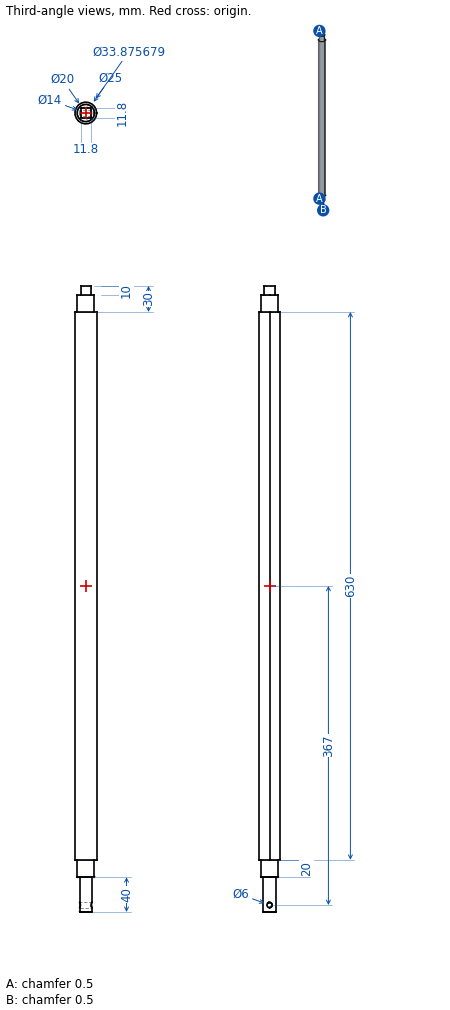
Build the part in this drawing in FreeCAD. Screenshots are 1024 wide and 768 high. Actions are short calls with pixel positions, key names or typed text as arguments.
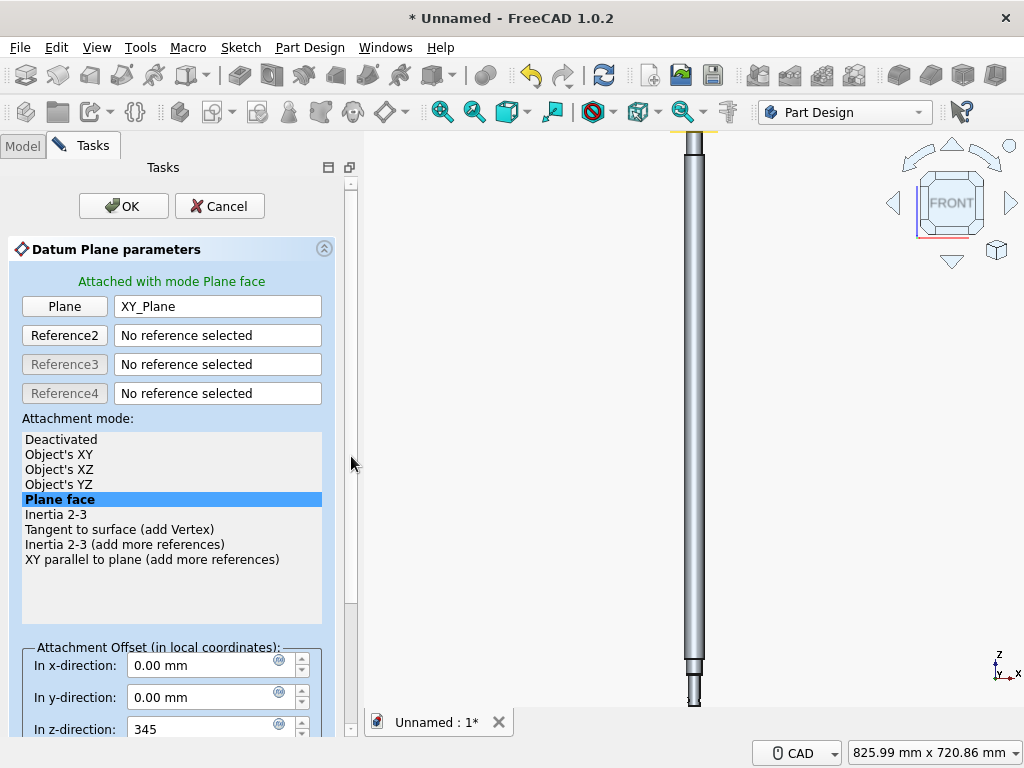
click(124, 206)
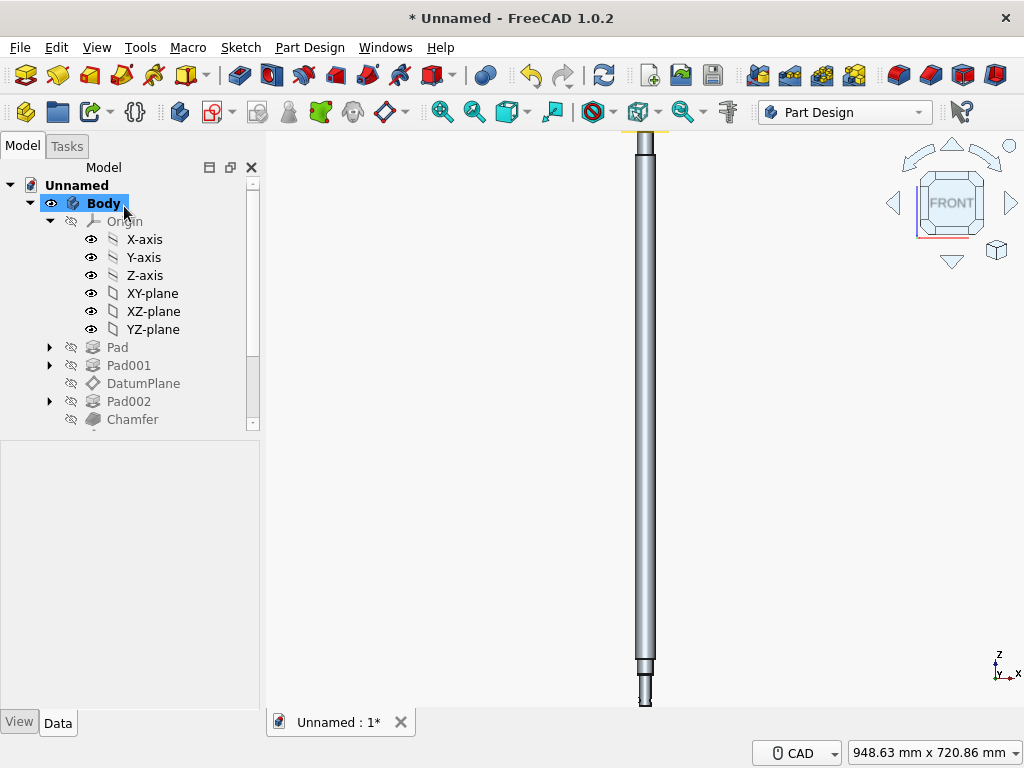
scroll(100, 307, down, 3)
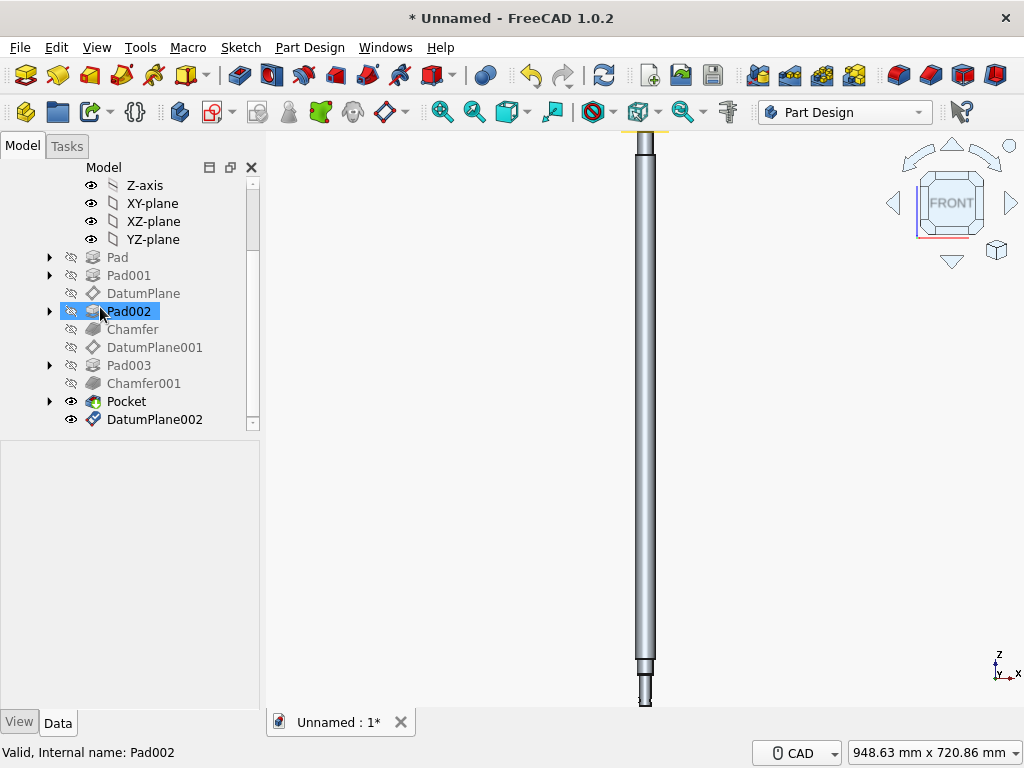
click(116, 419)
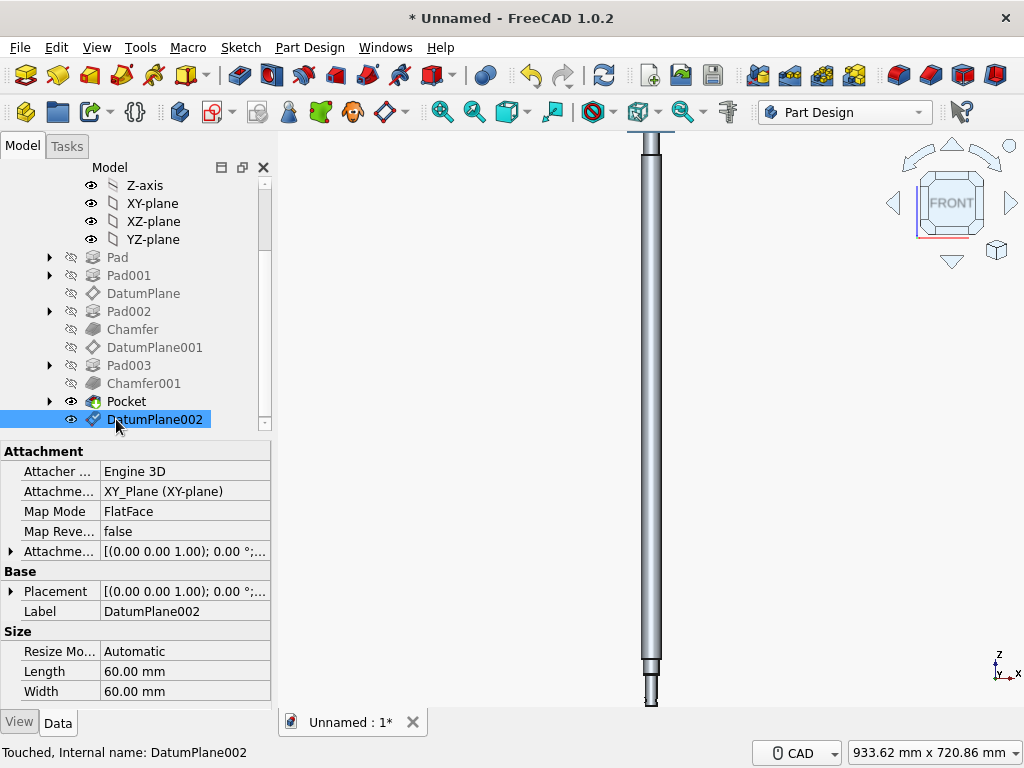
click(212, 112)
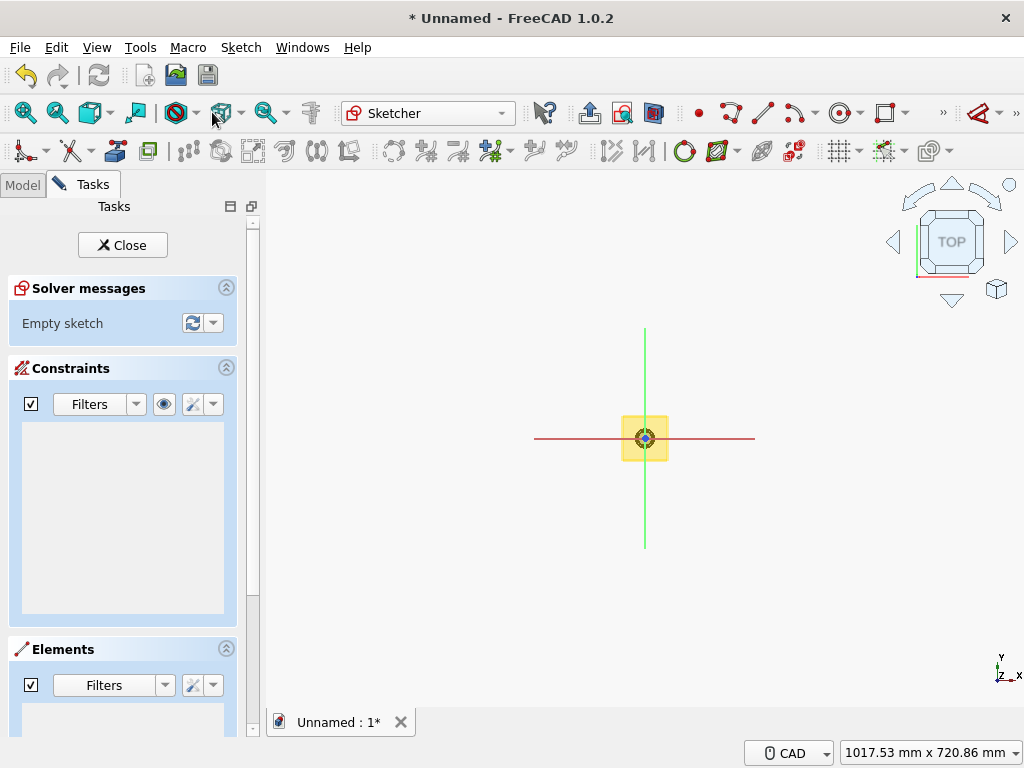
scroll(650, 438, up, 13)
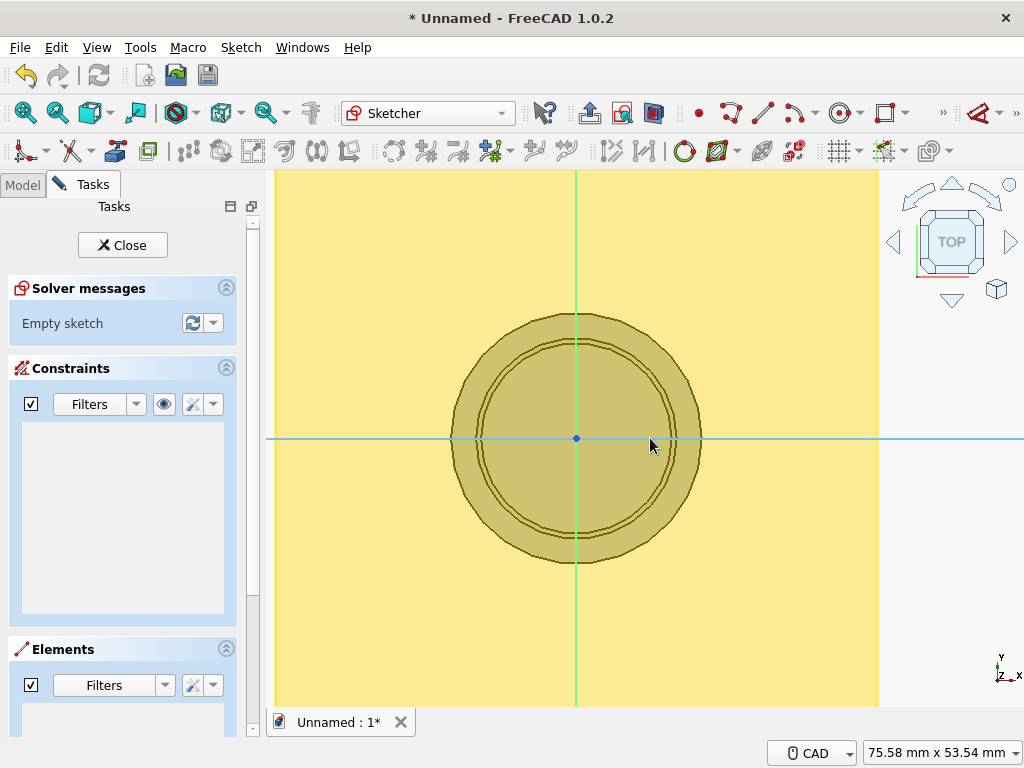
click(908, 114)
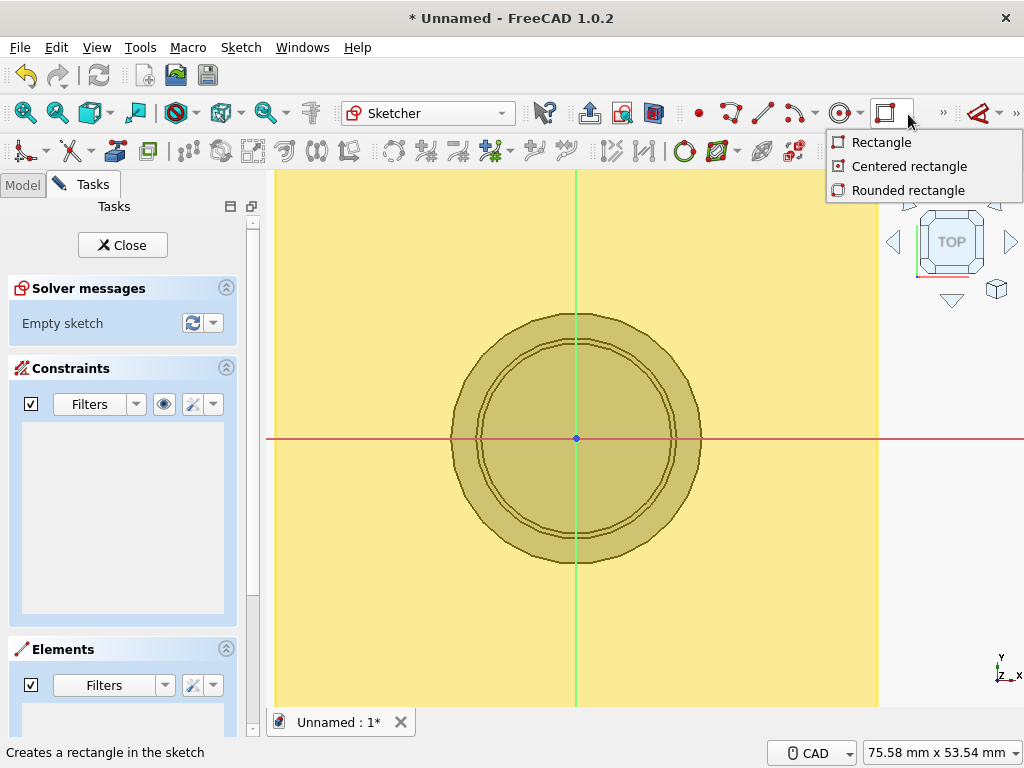
click(924, 166)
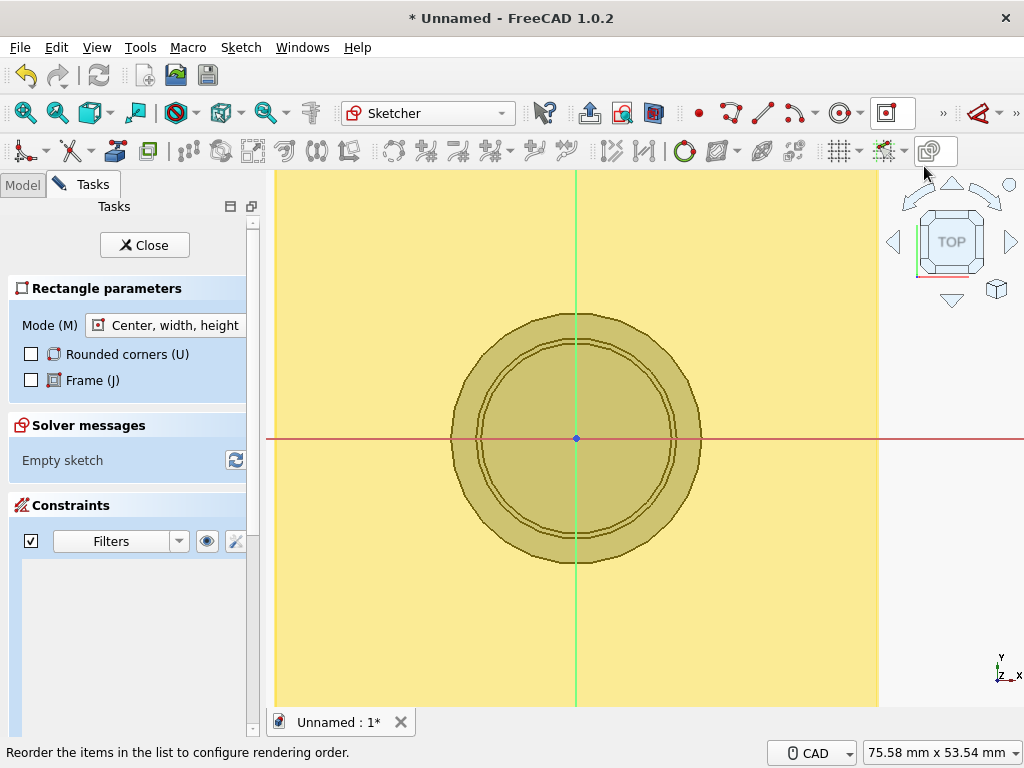
click(576, 438)
move(636, 379)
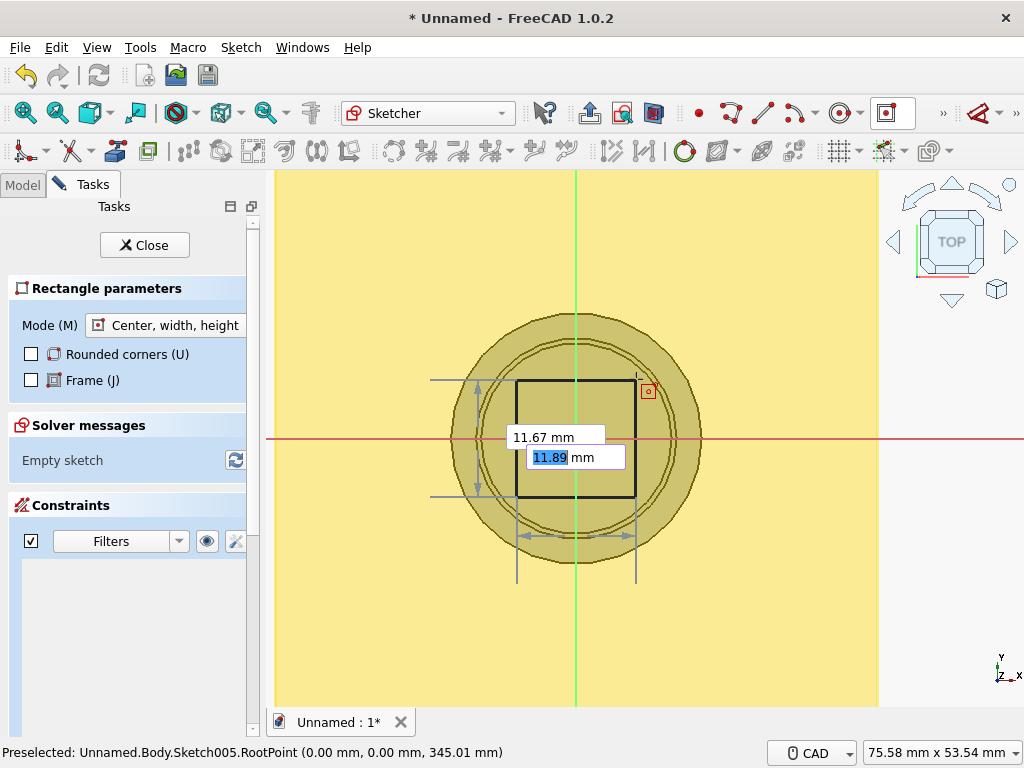
text(11.8)
key(Tab)
text(11.8)
key(Return)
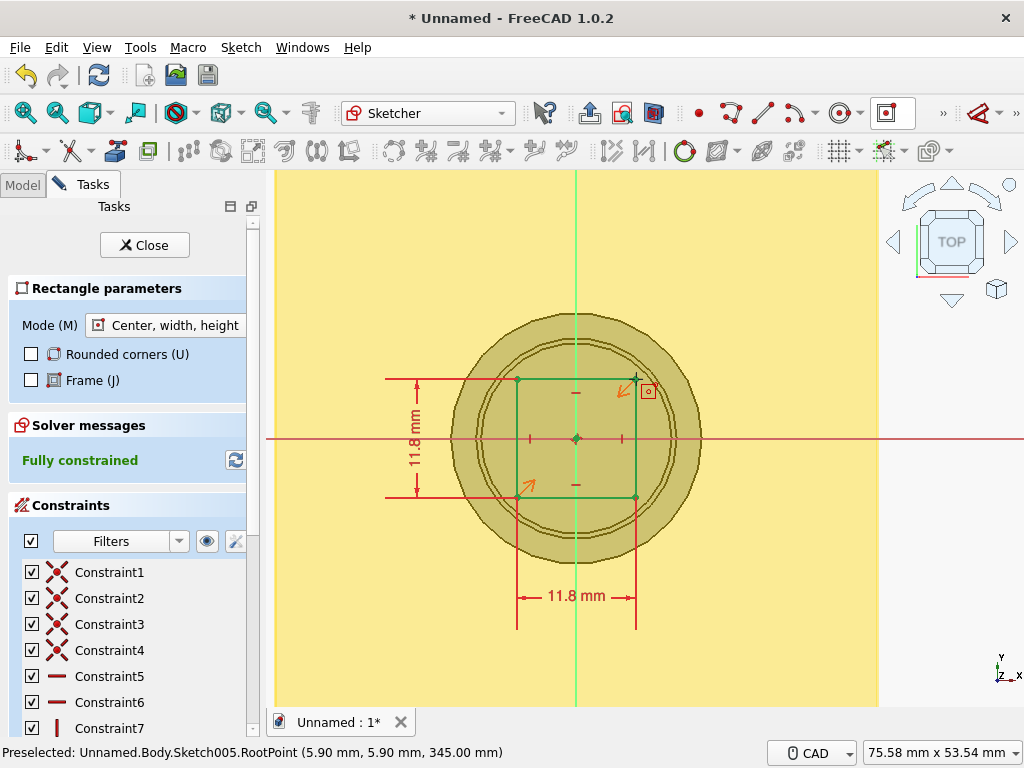
click(840, 114)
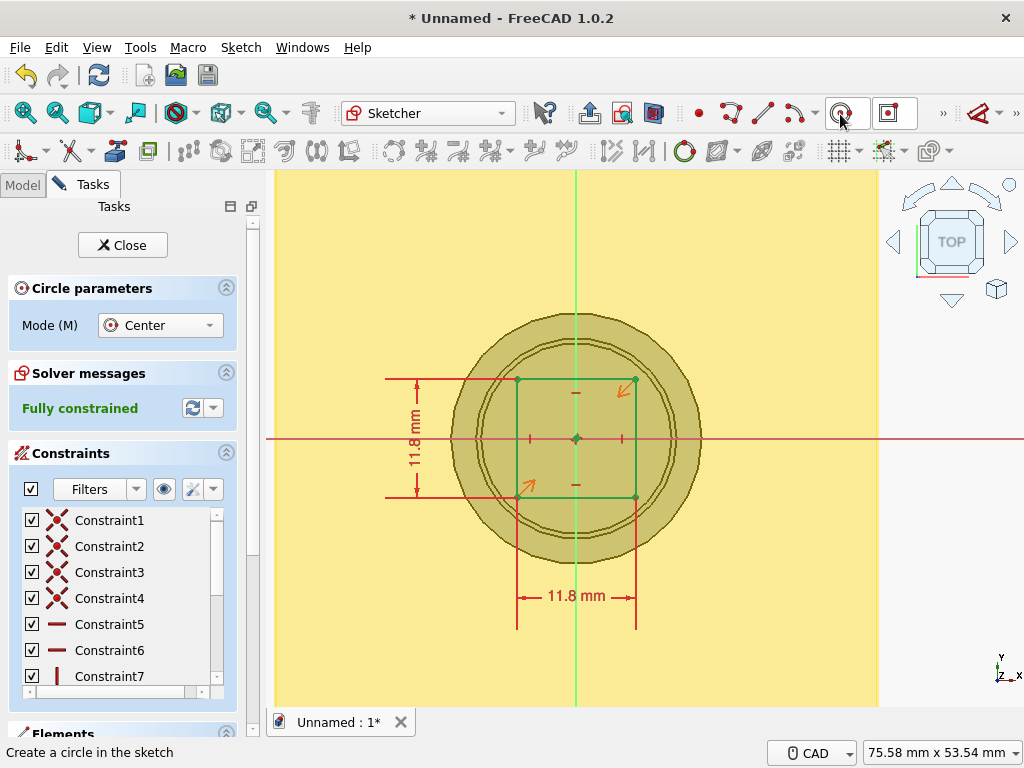
click(576, 438)
move(696, 318)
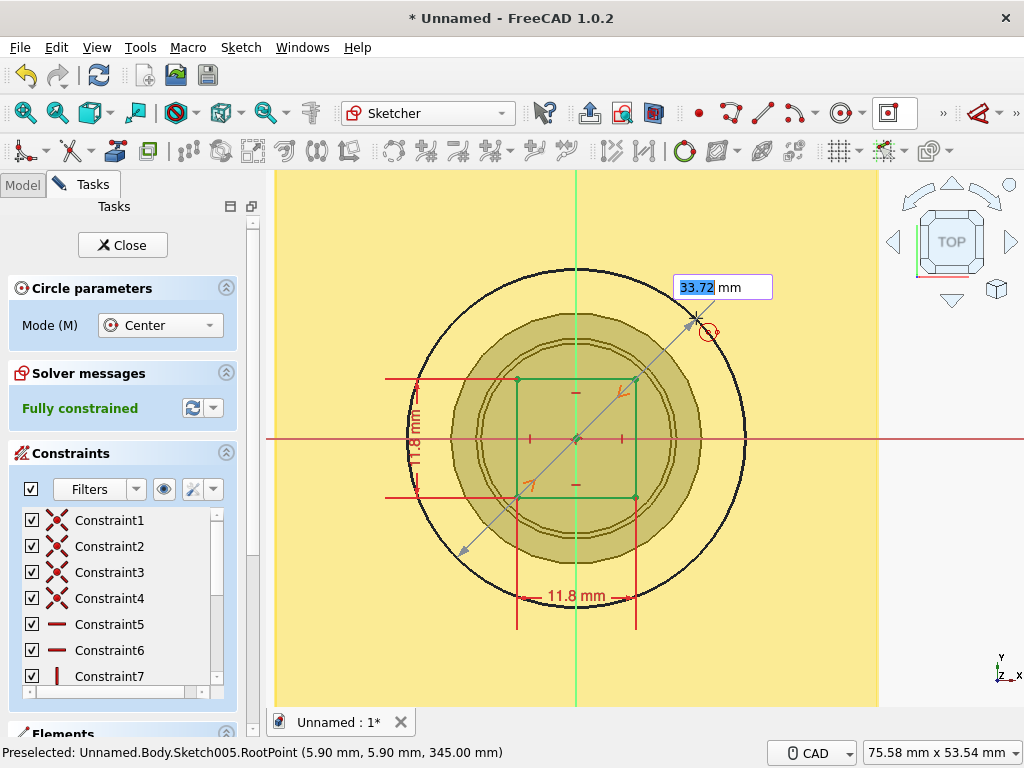
text(33.875679)
key(Return)
key(Escape)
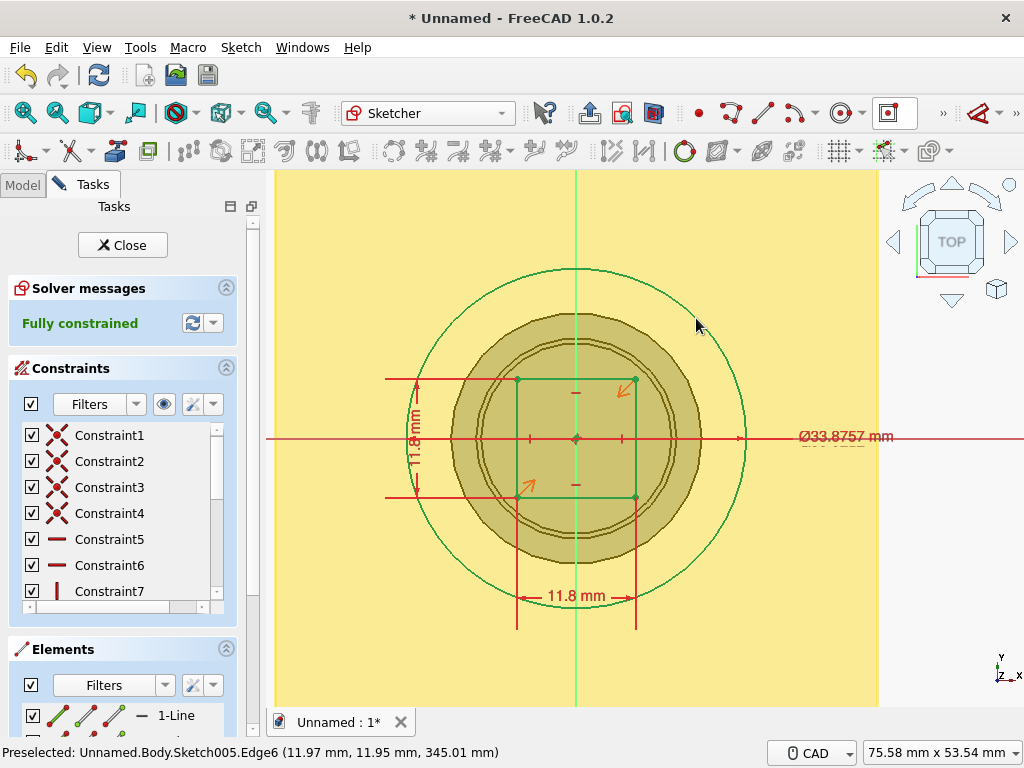
click(123, 245)